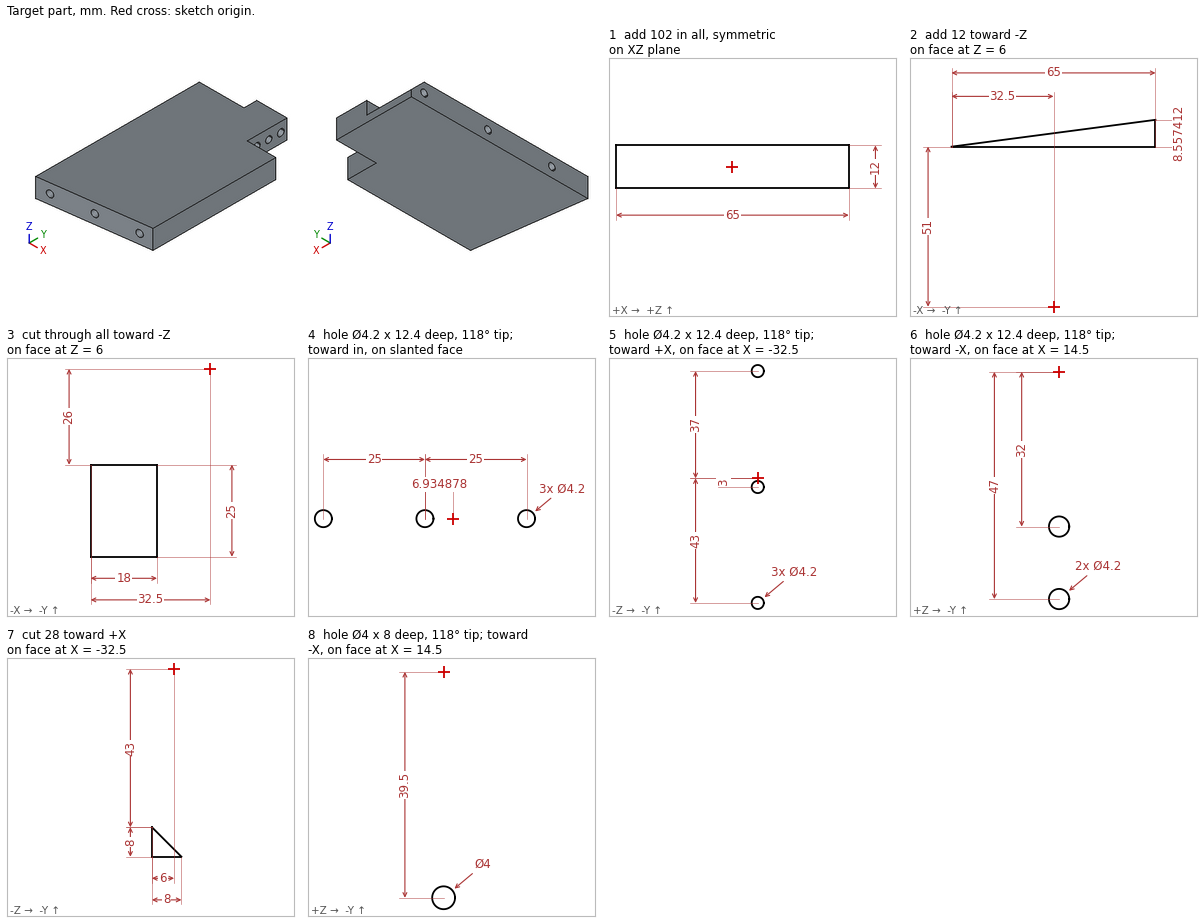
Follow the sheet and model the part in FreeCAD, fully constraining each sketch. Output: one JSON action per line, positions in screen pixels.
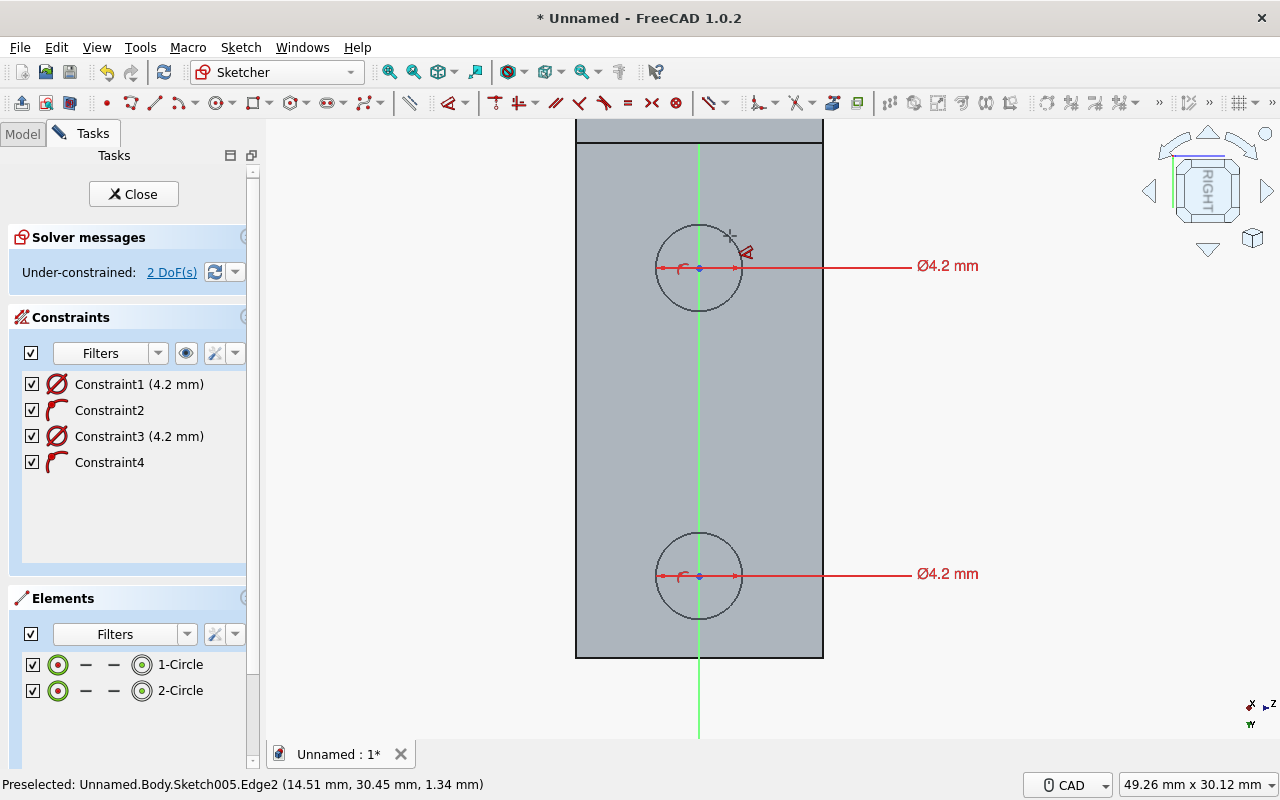
{"action": "left_click", "coordinate": [699, 576]}
{"action": "left_click", "coordinate": [733, 362]}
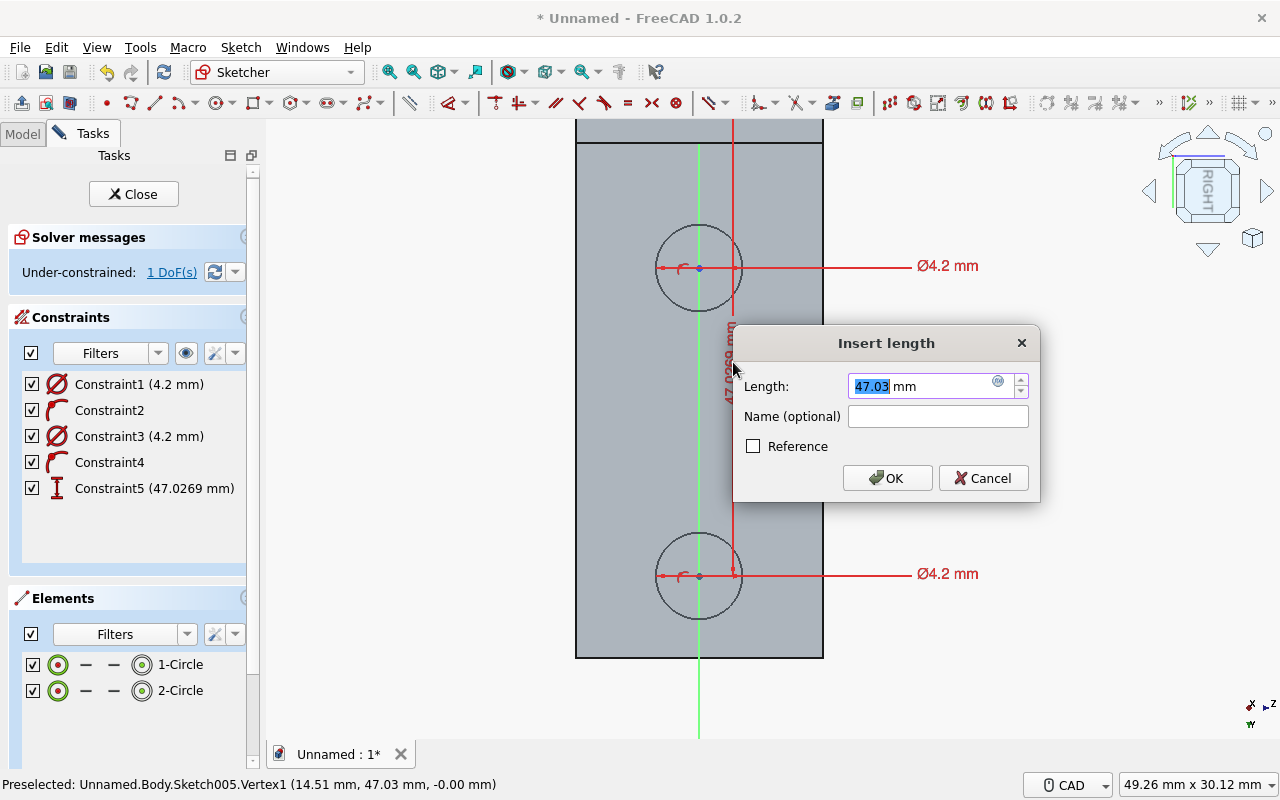
{"action": "type", "text": "47"}
{"action": "key", "text": "Return"}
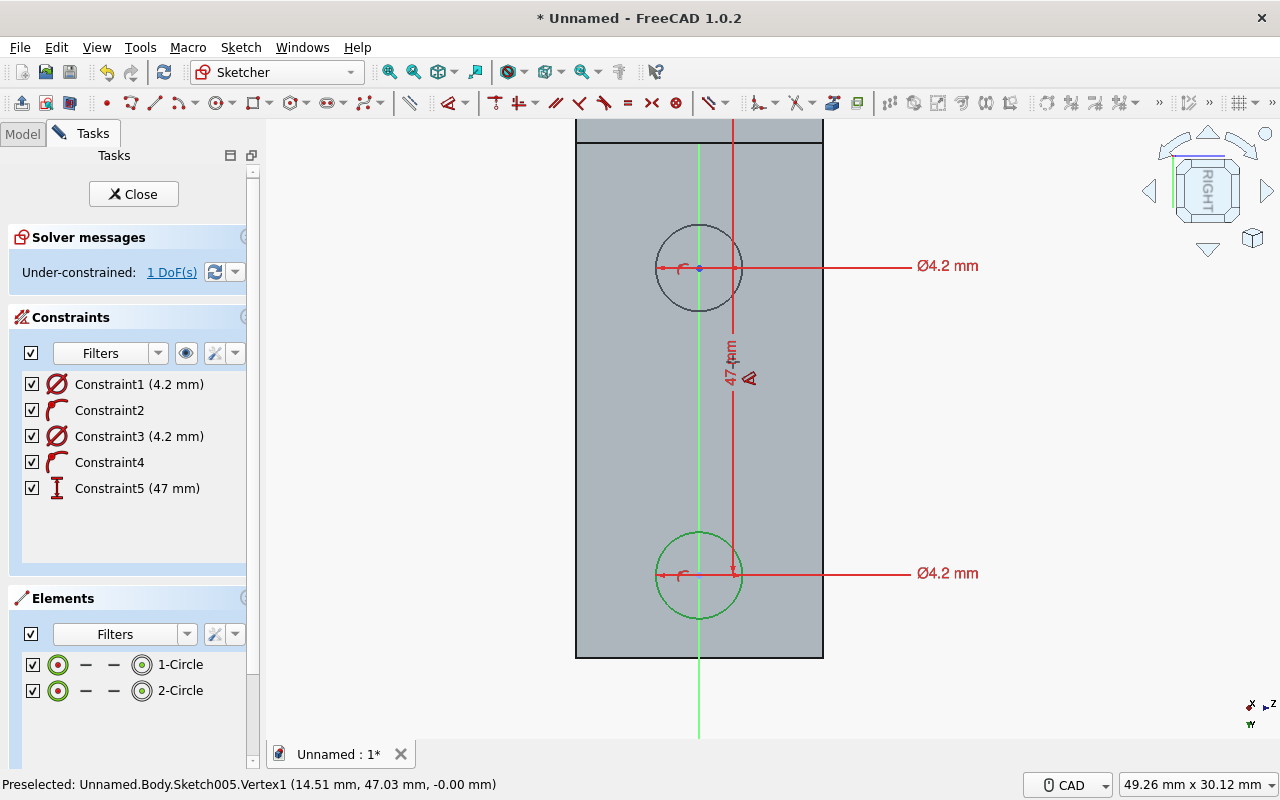
{"action": "left_click", "coordinate": [699, 268]}
{"action": "left_click", "coordinate": [733, 207]}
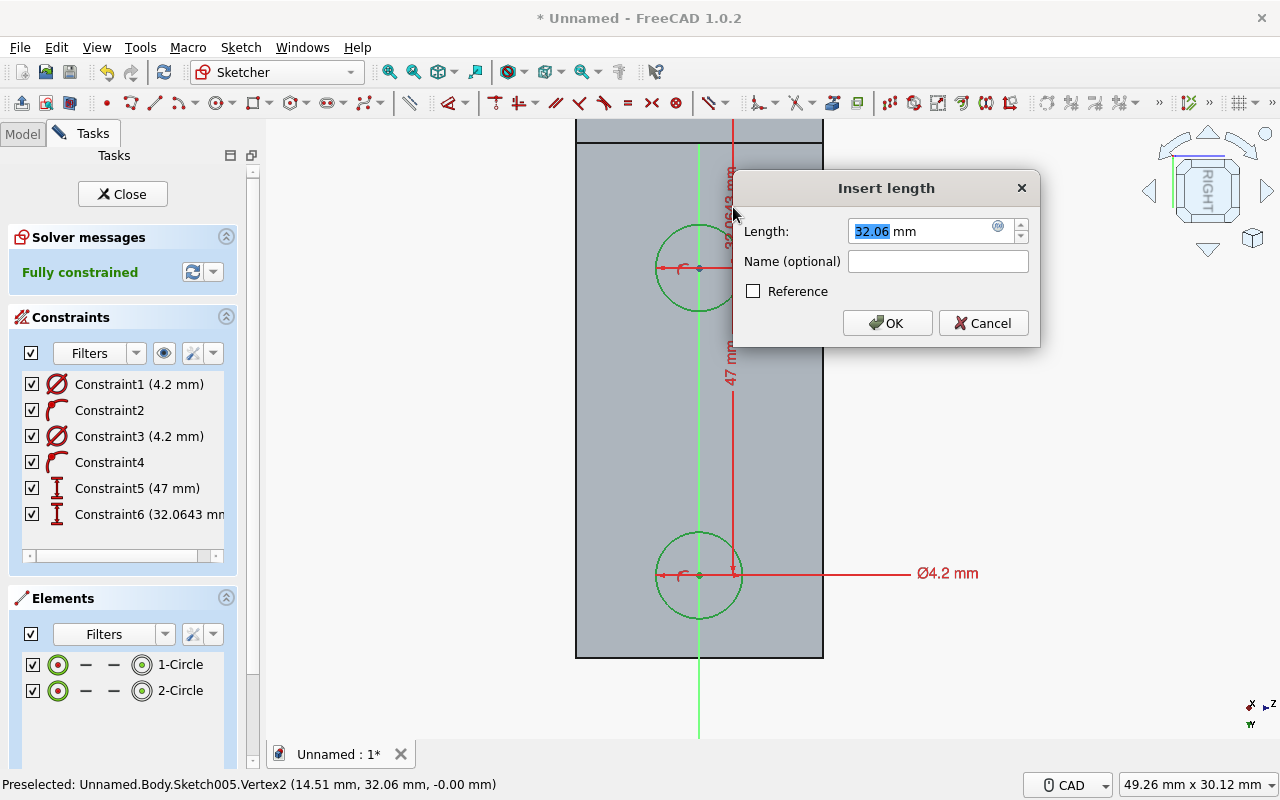
{"action": "type", "text": "32"}
{"action": "key", "text": "Return"}
{"action": "key", "text": "Escape"}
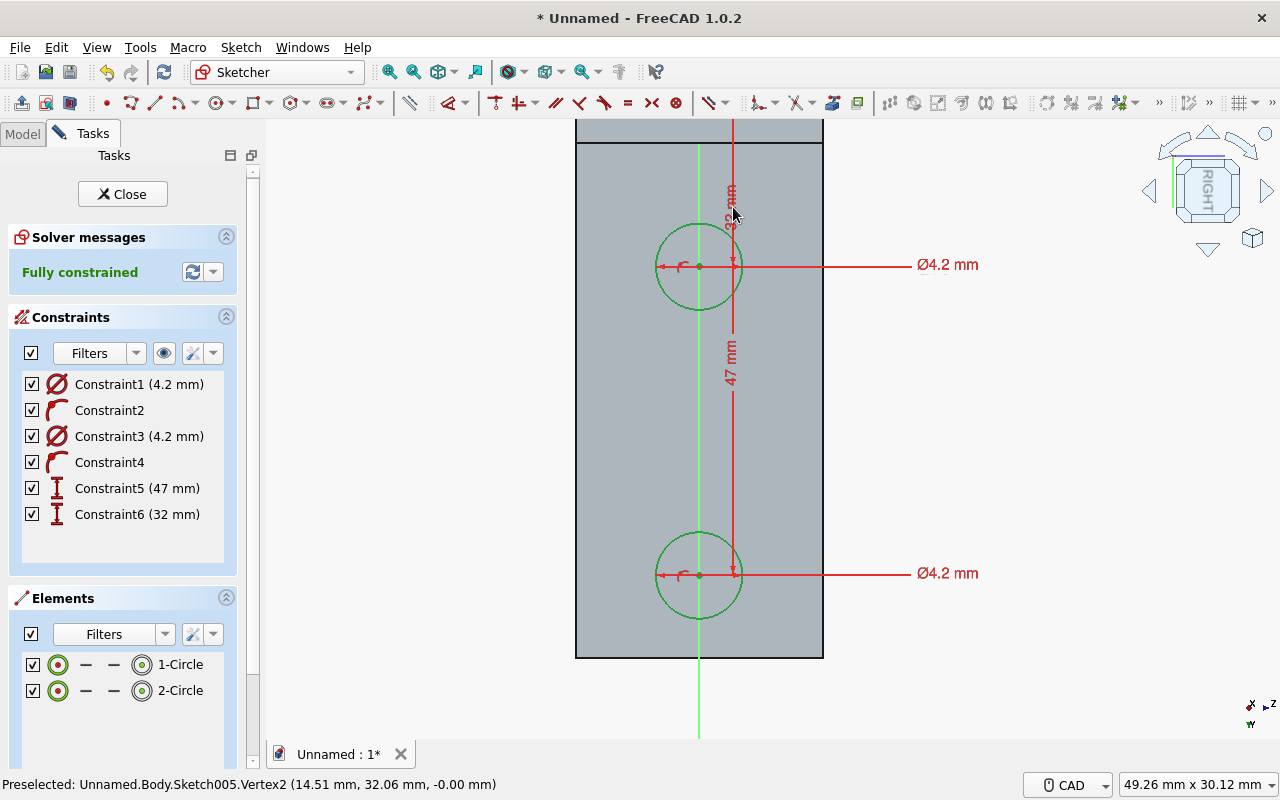
{"action": "left_click", "coordinate": [123, 194]}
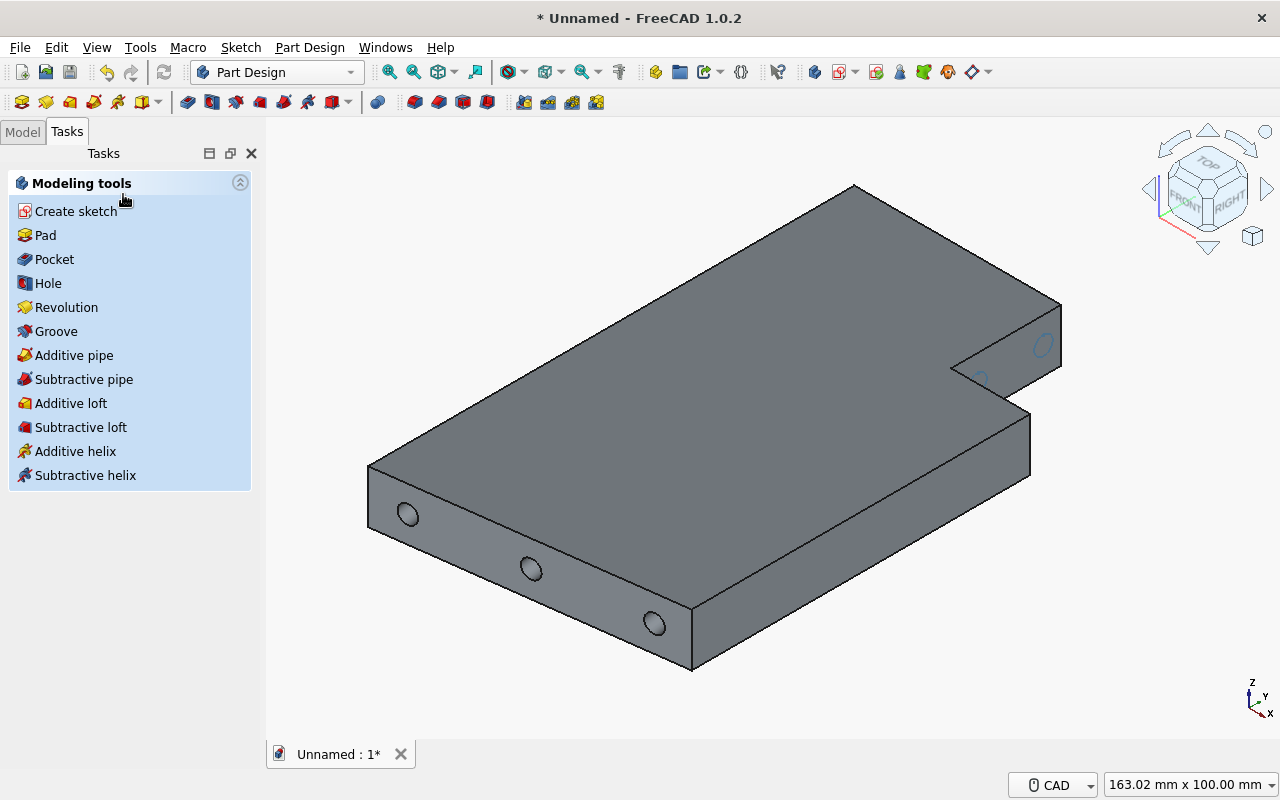
{"action": "left_click", "coordinate": [212, 102]}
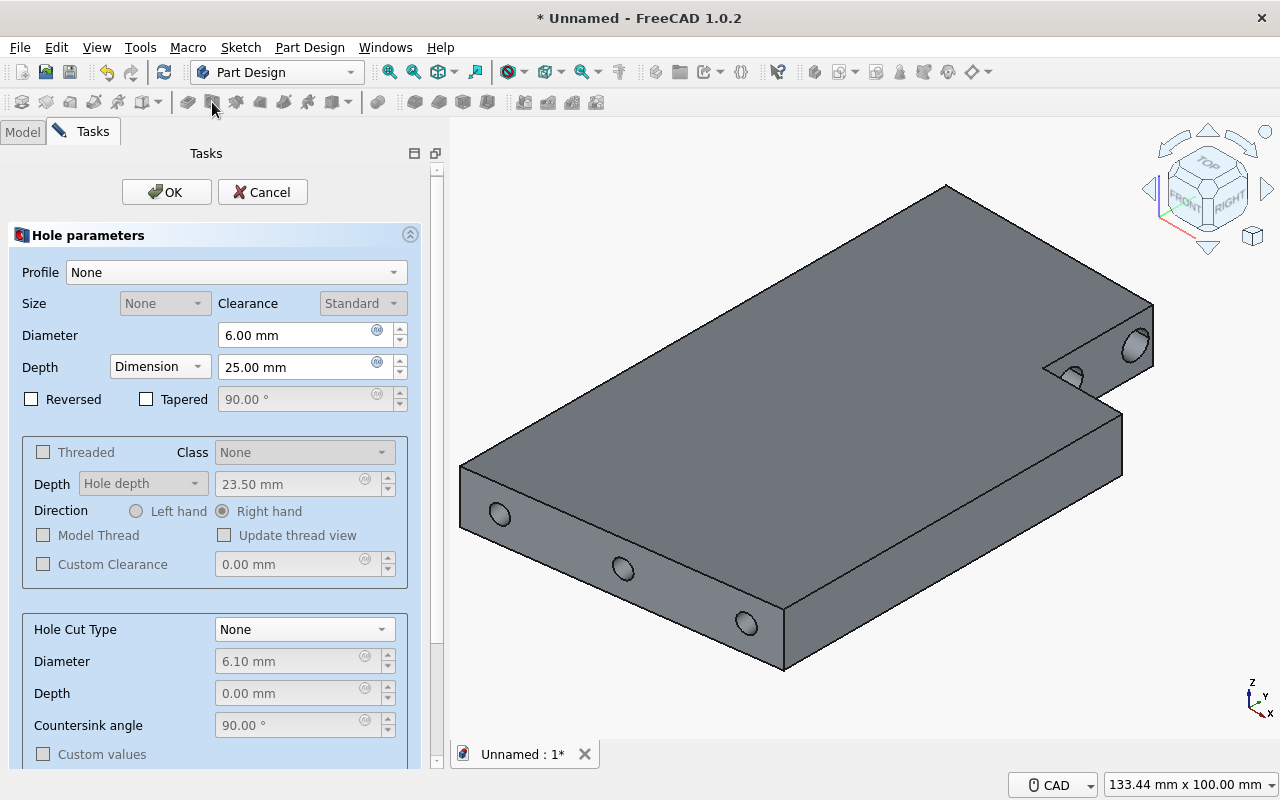
{"action": "triple_click", "coordinate": [305, 335]}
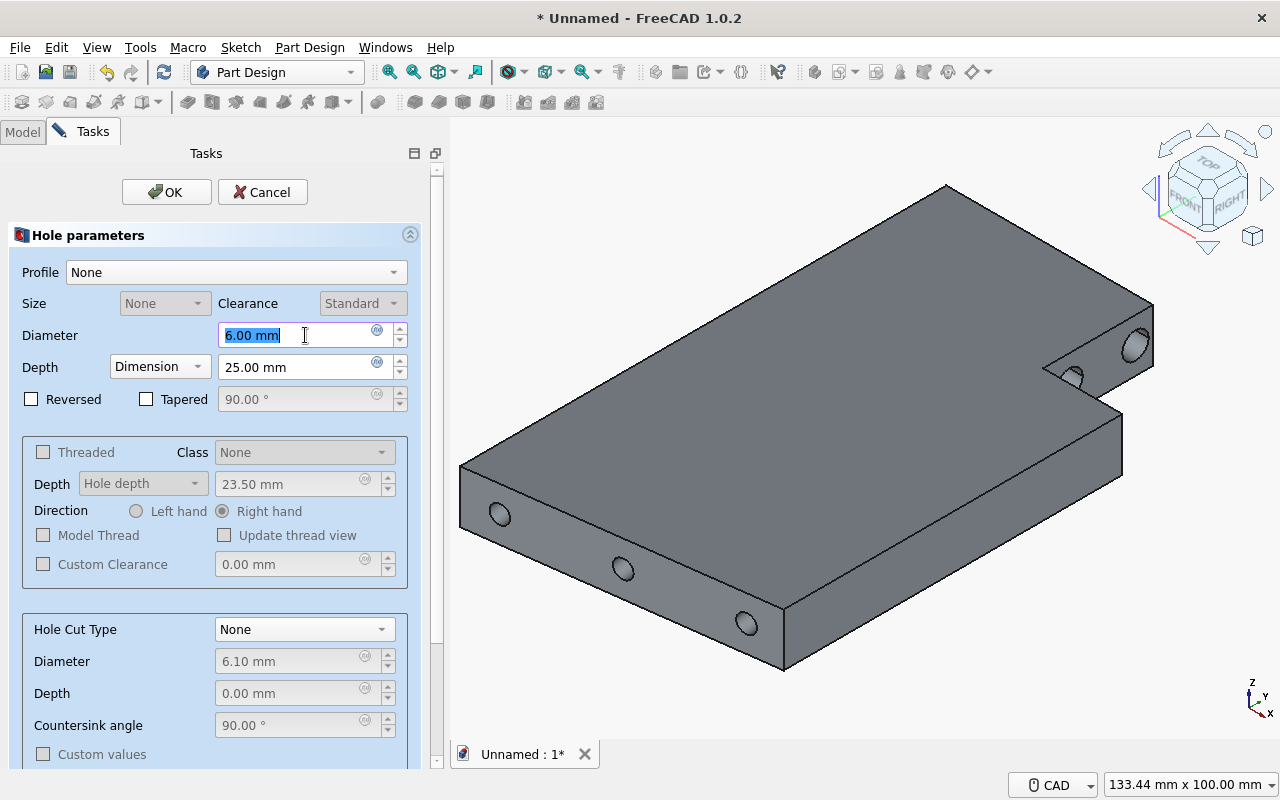
{"action": "type", "text": "4.2"}
{"action": "key", "text": "Tab"}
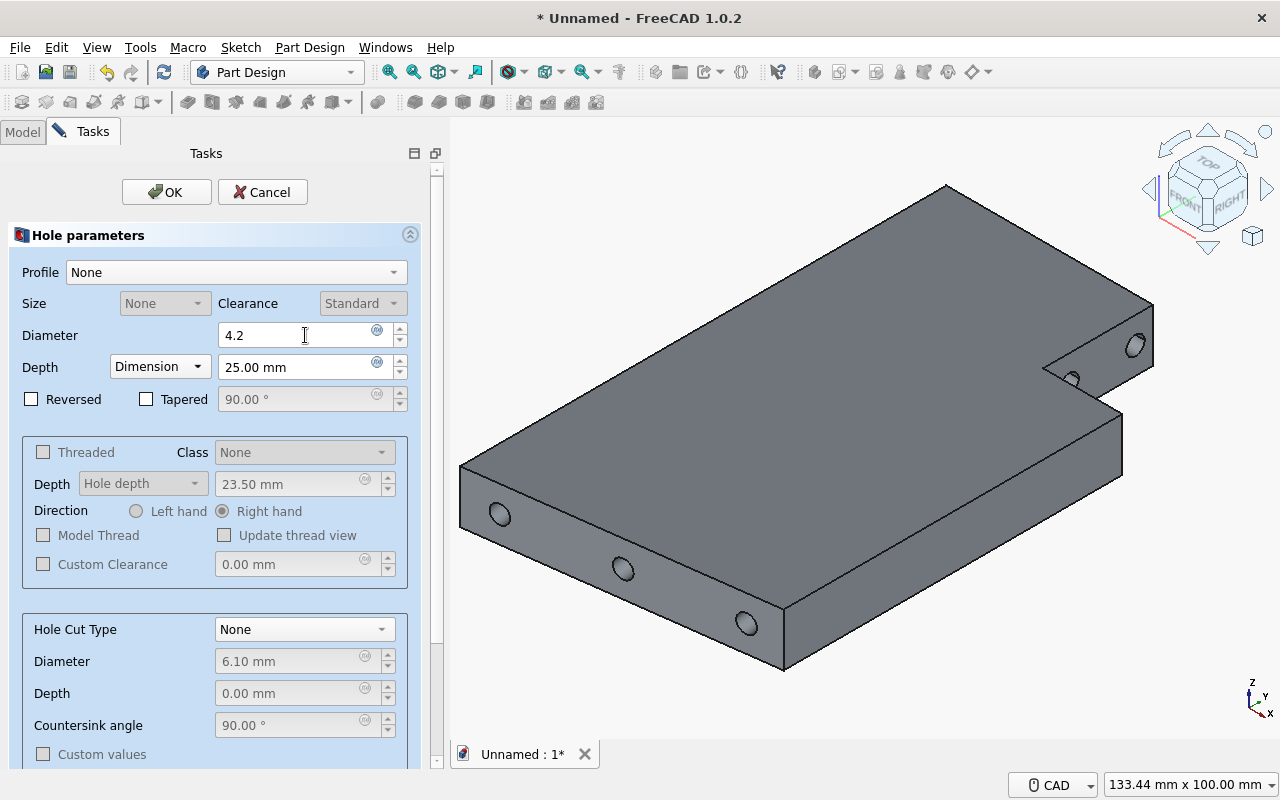
{"action": "triple_click", "coordinate": [305, 367]}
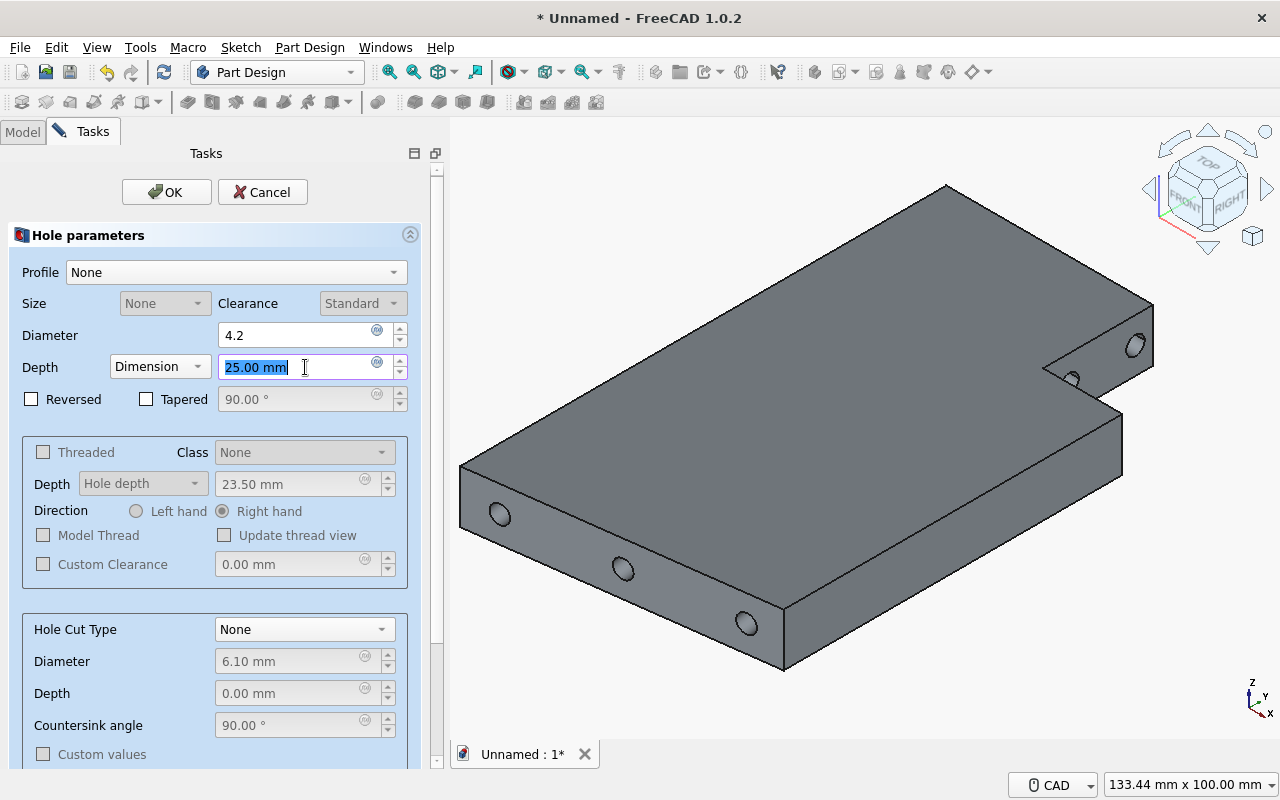
{"action": "type", "text": "12.4"}
{"action": "key", "text": "Tab"}